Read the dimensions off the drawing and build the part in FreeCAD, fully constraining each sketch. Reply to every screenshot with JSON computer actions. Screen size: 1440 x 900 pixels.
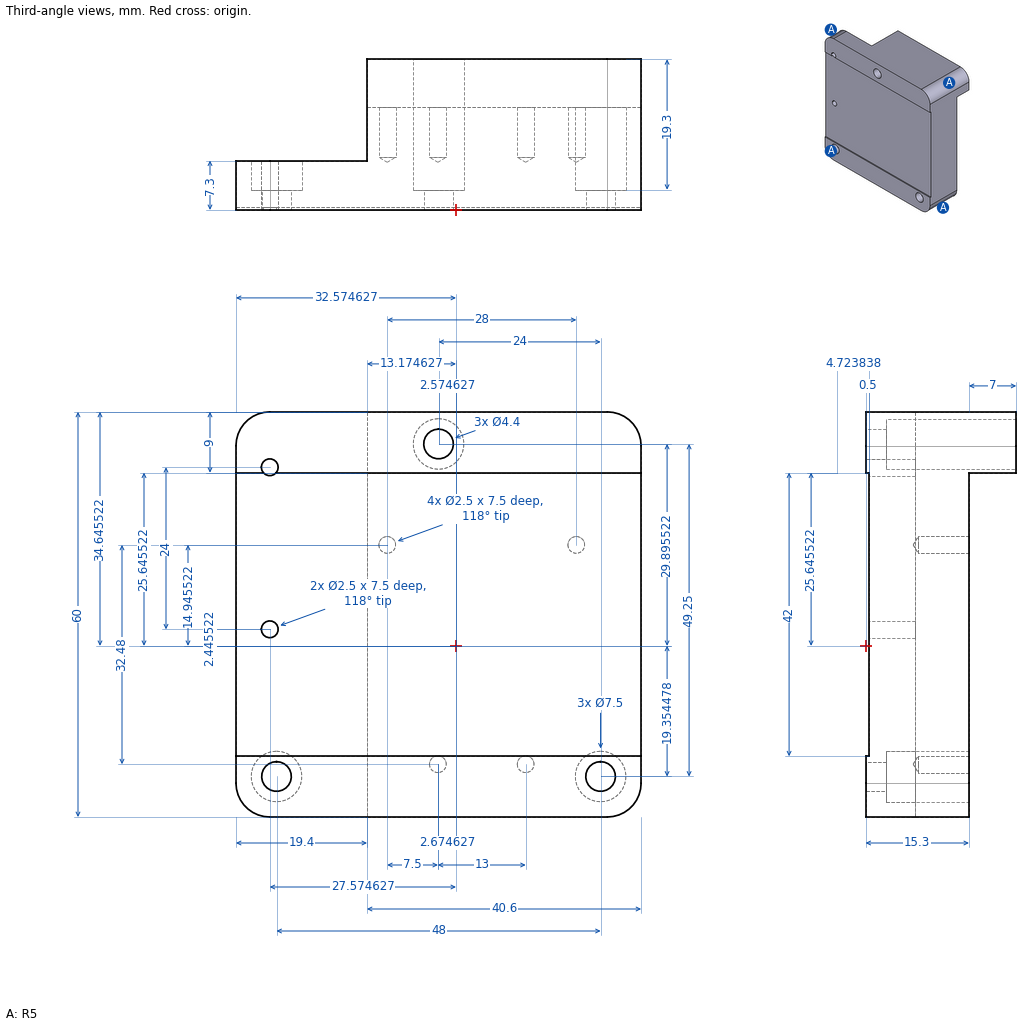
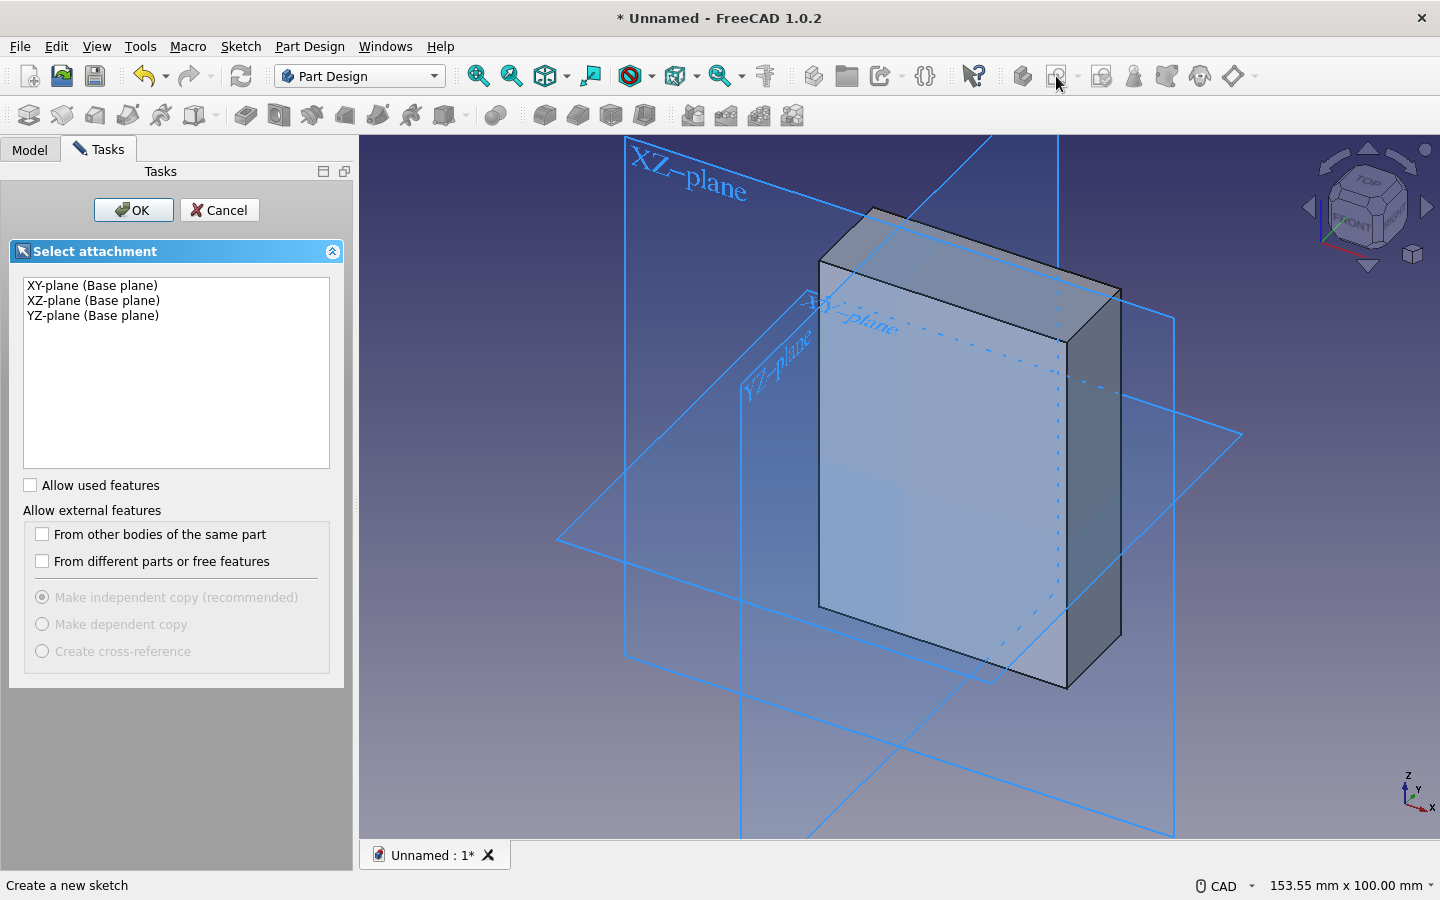
{"action": "left_click", "coordinate": [84, 300]}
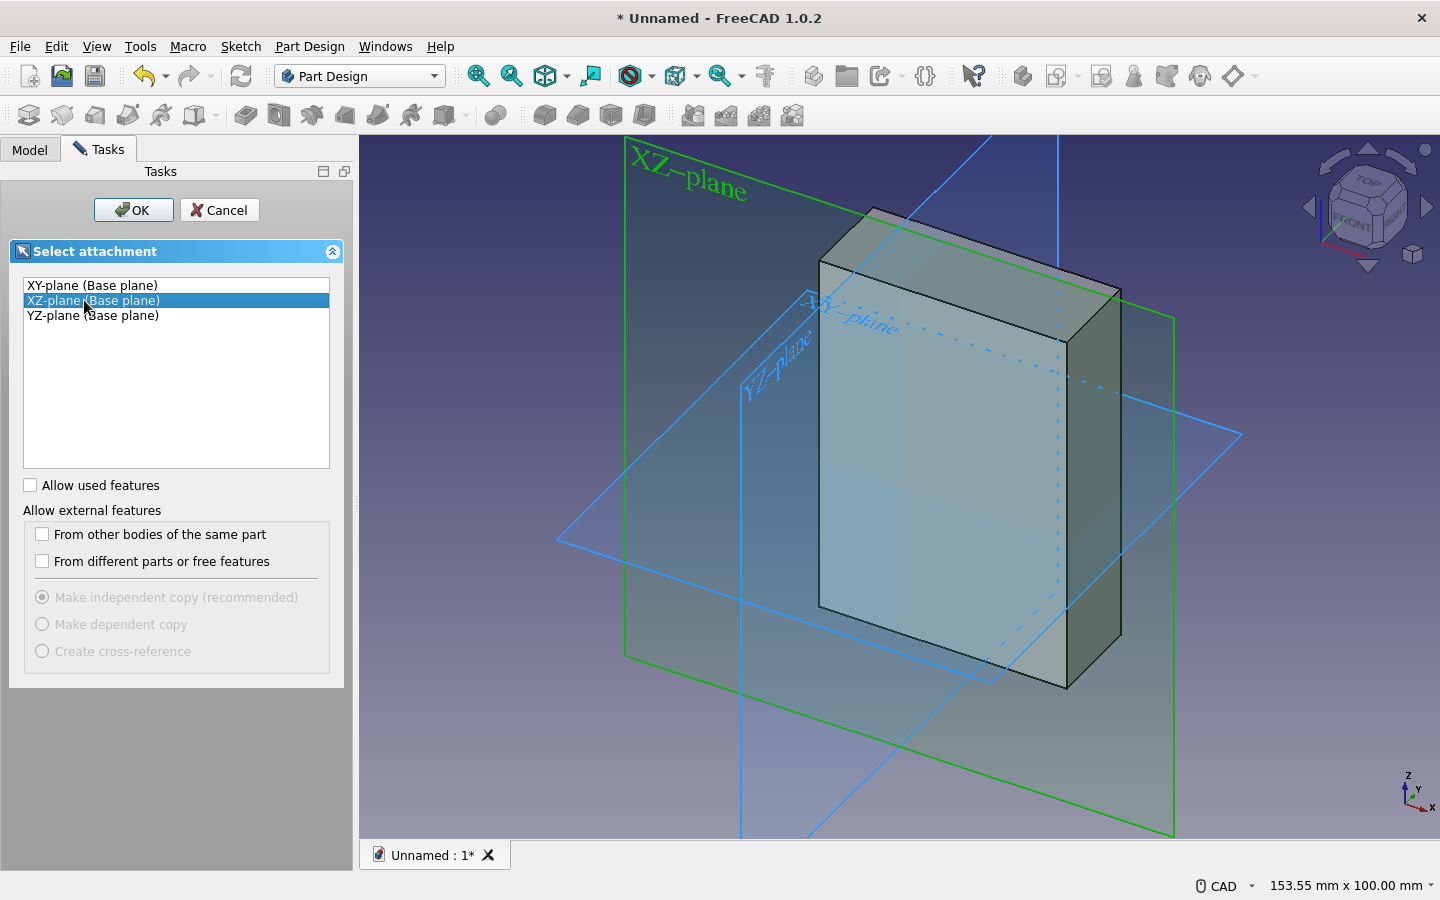
{"action": "left_click", "coordinate": [134, 210]}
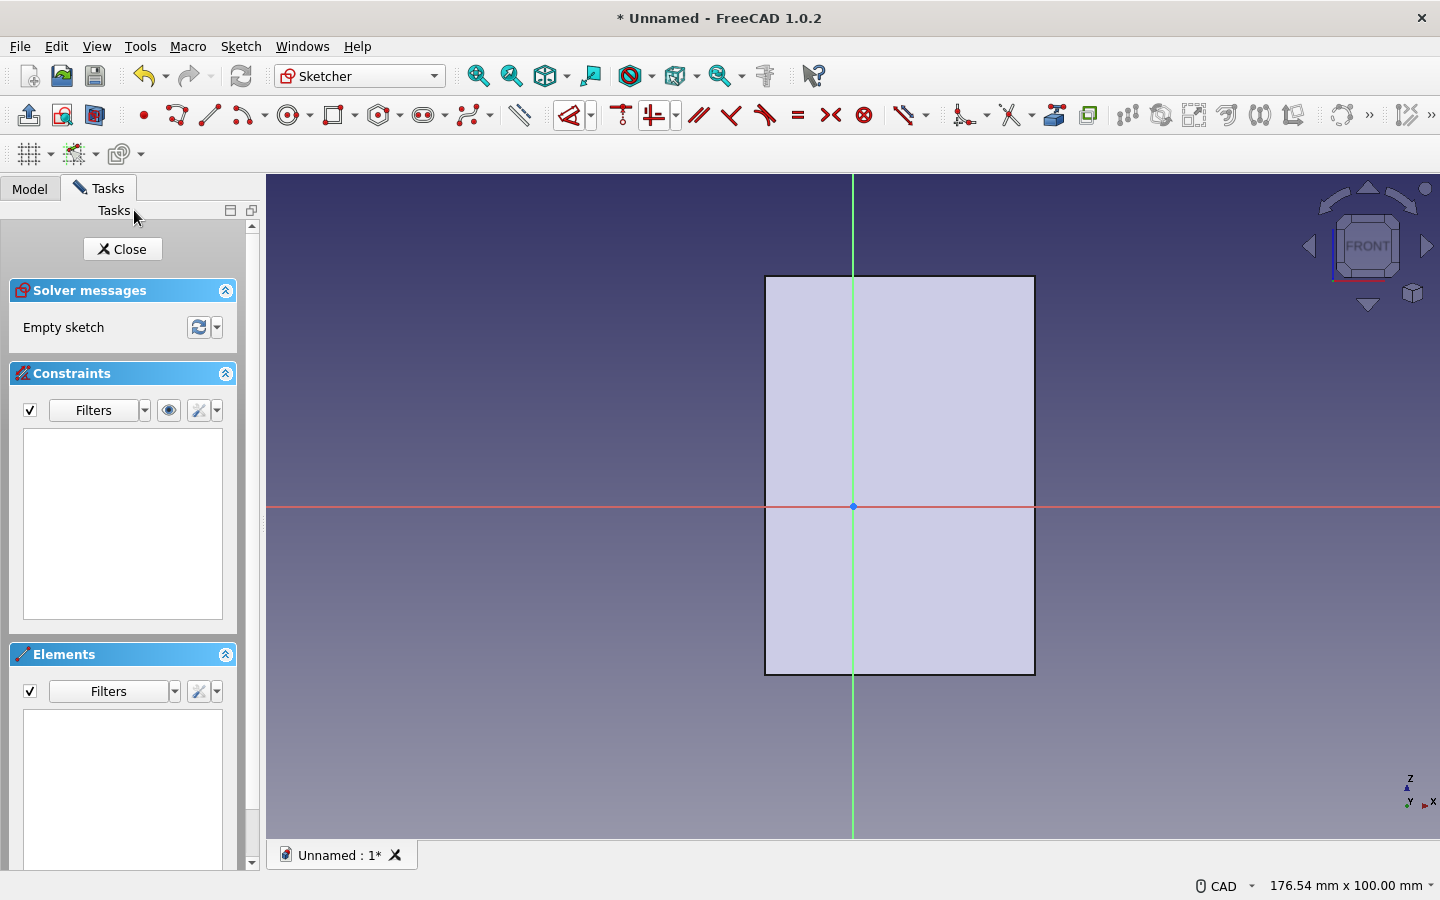
{"action": "key", "text": "g r"}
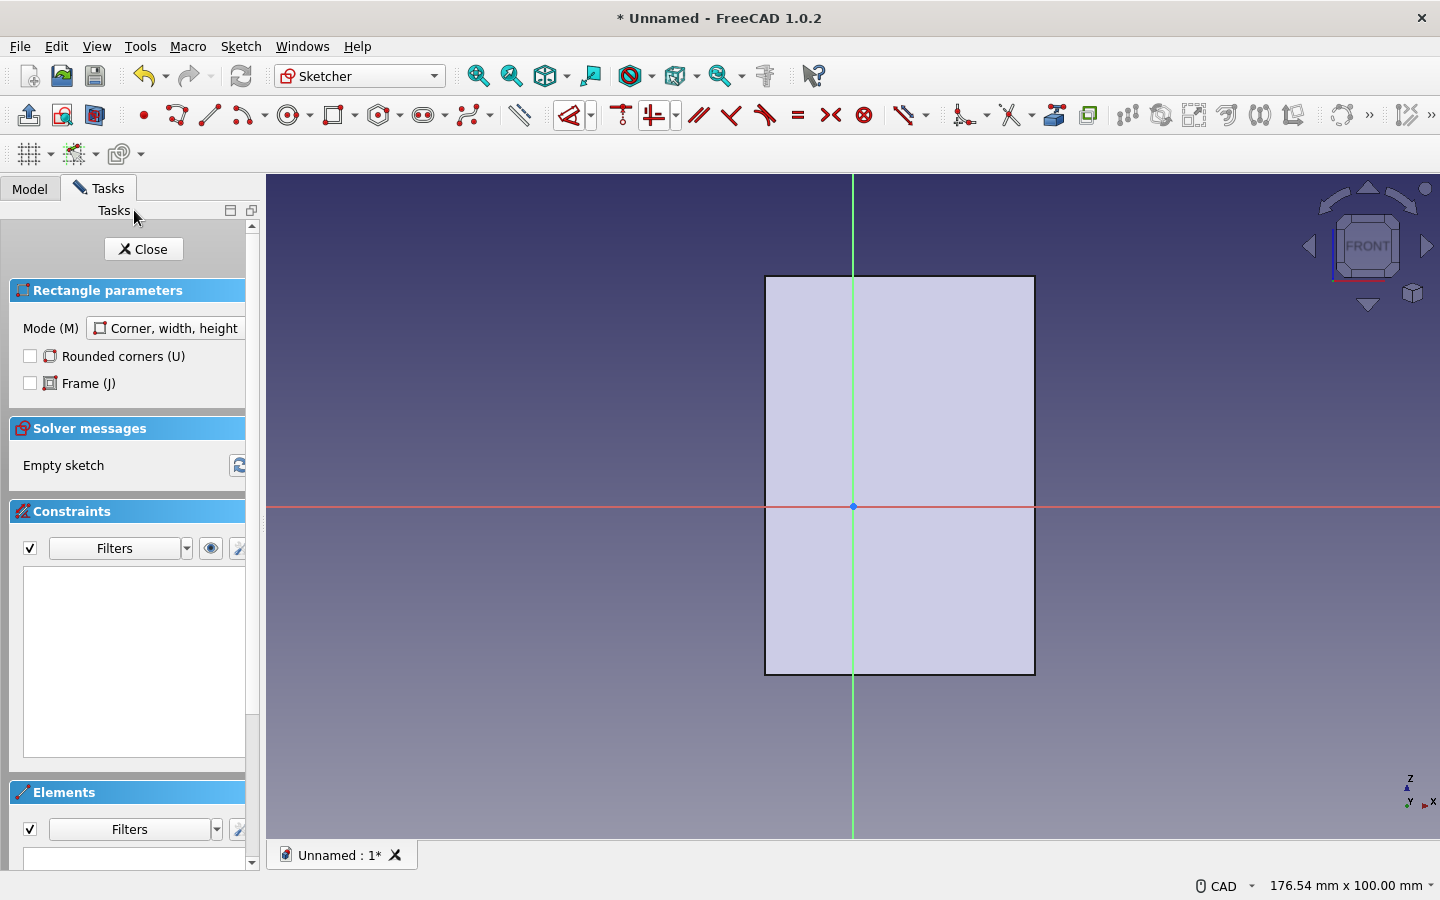
{"action": "left_click", "coordinate": [636, 276]}
{"action": "left_click", "coordinate": [765, 675]}
{"action": "key", "text": "Escape"}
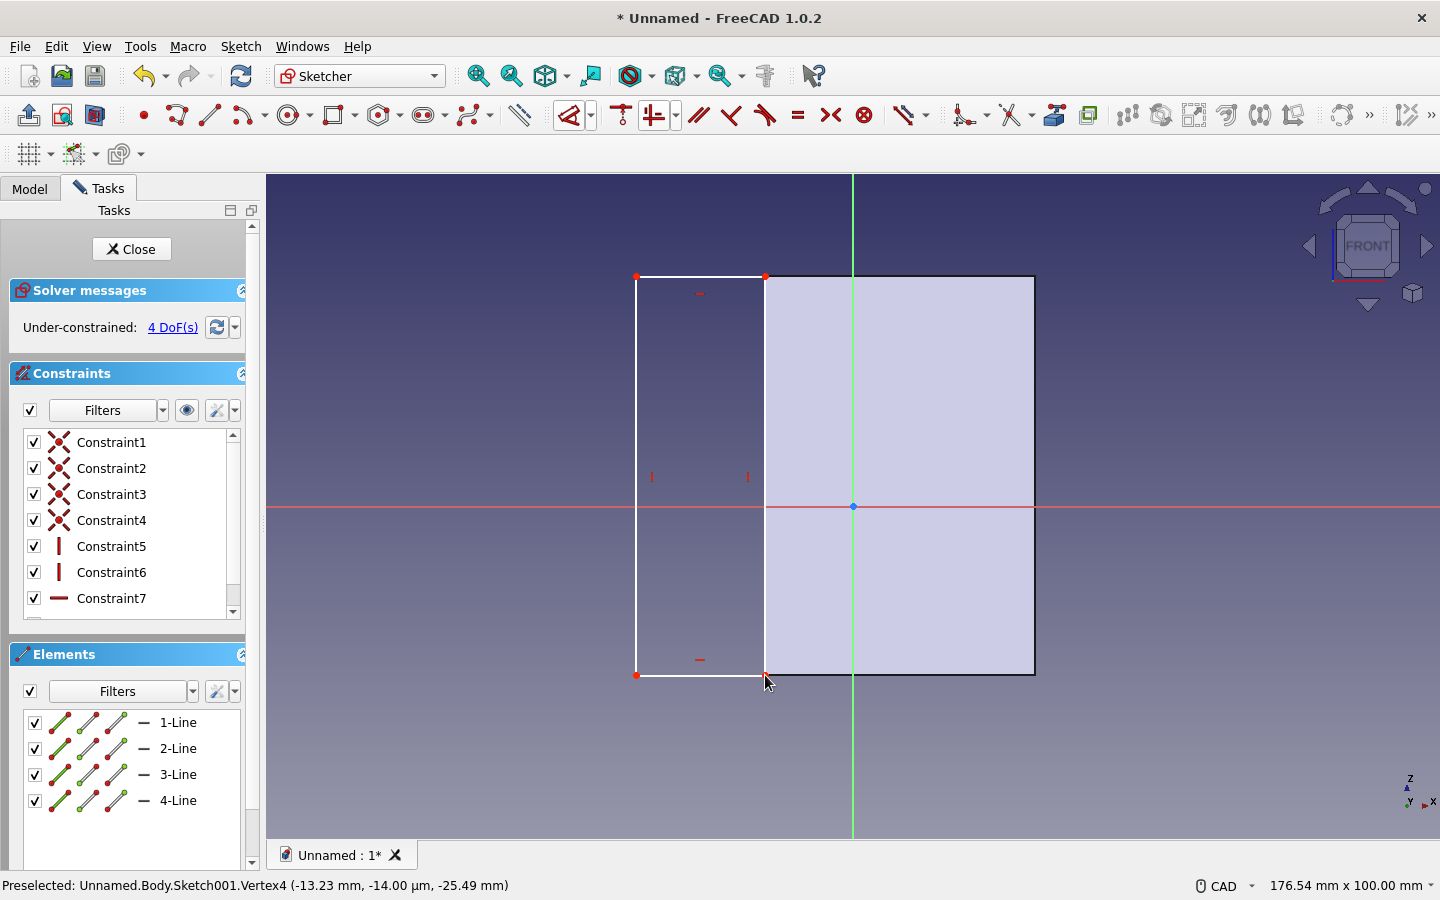
{"action": "key", "text": "d"}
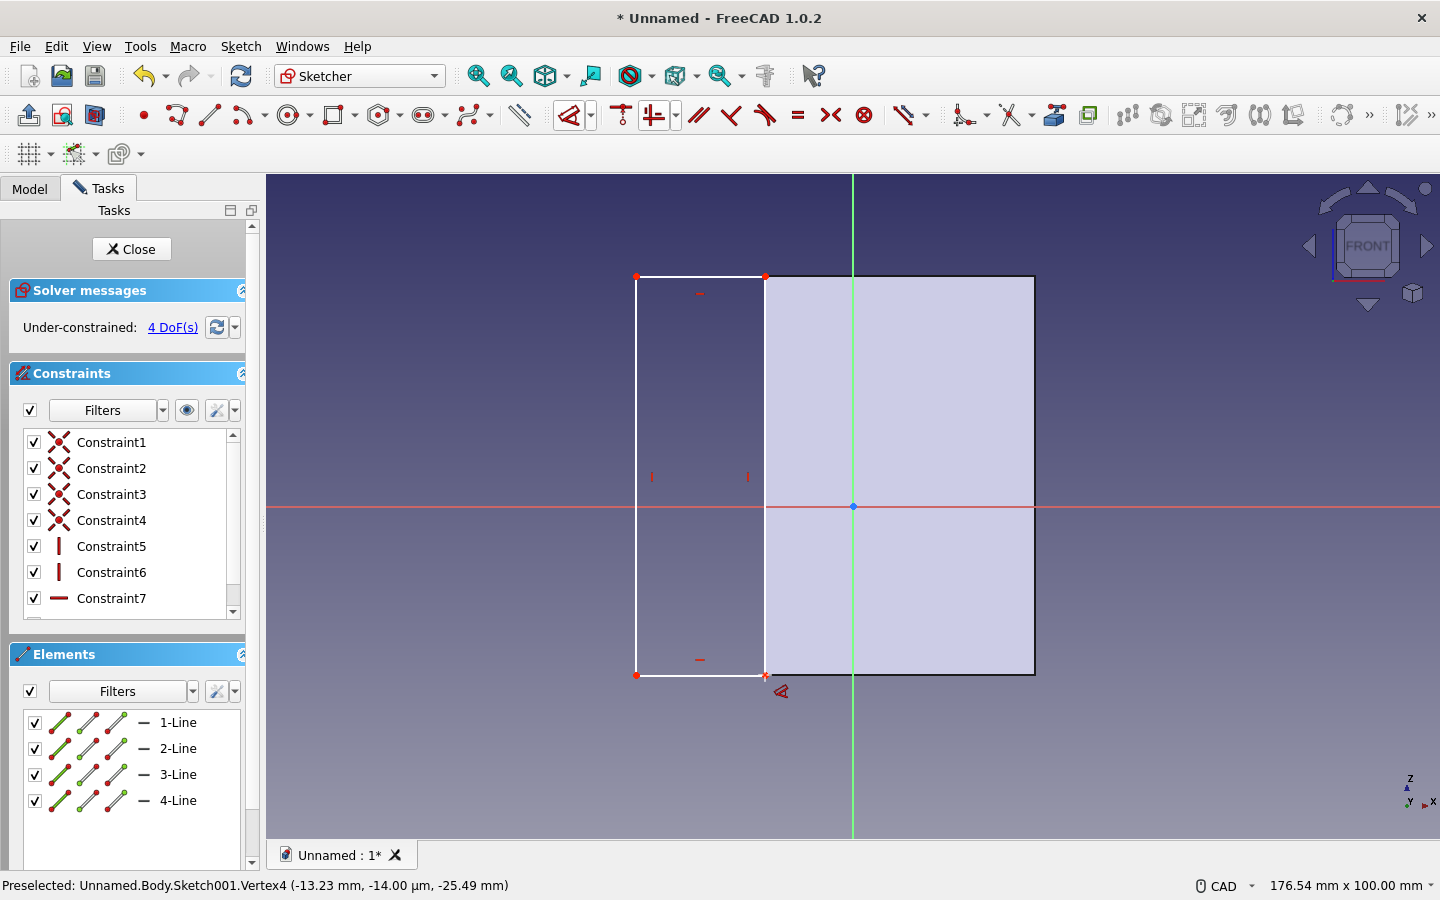
{"action": "left_click", "coordinate": [636, 397]}
{"action": "left_click", "coordinate": [602, 476]}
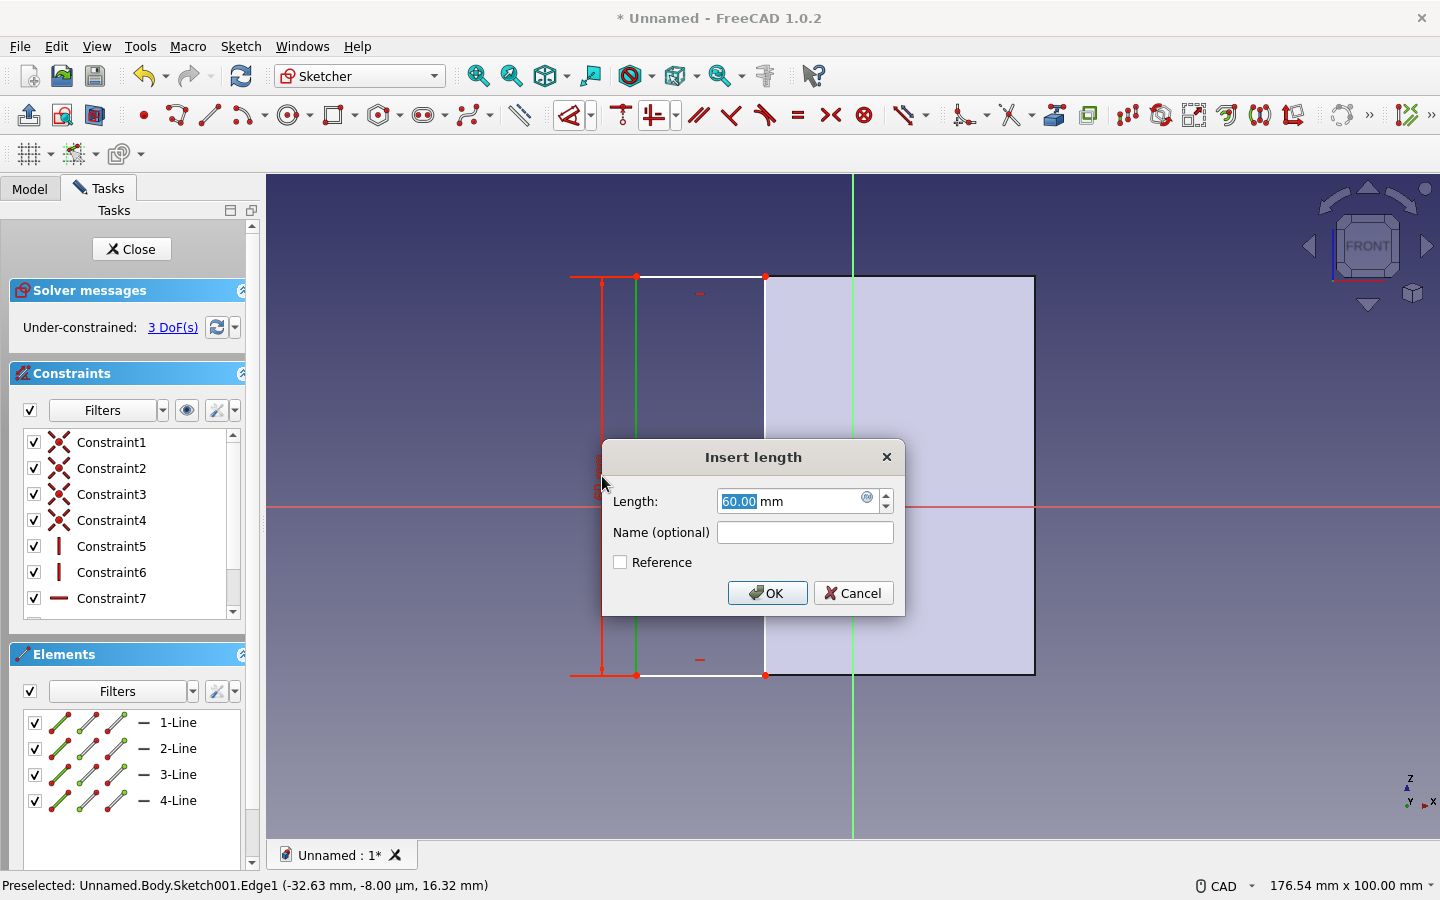
{"action": "type", "text": "60"}
{"action": "key", "text": "Return"}